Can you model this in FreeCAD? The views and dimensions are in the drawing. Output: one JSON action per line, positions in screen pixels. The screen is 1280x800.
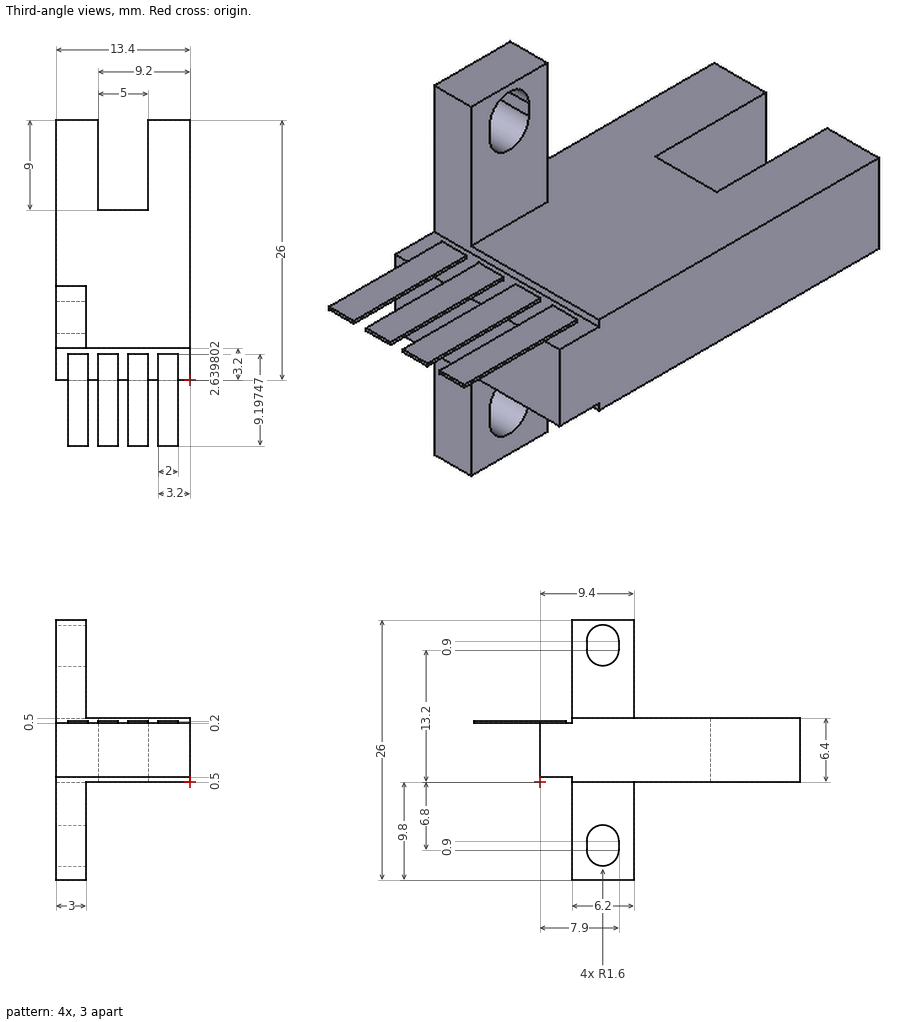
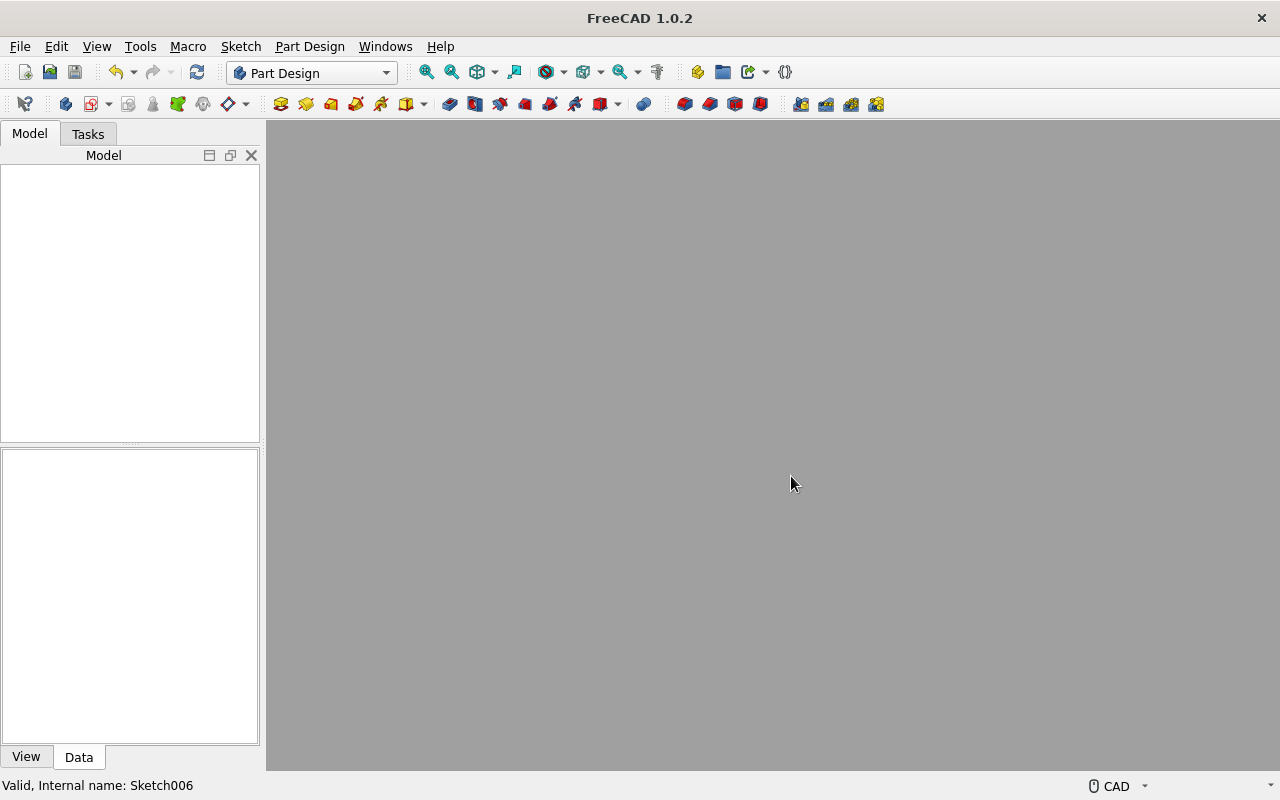
{"action": "left_click", "coordinate": [25, 72]}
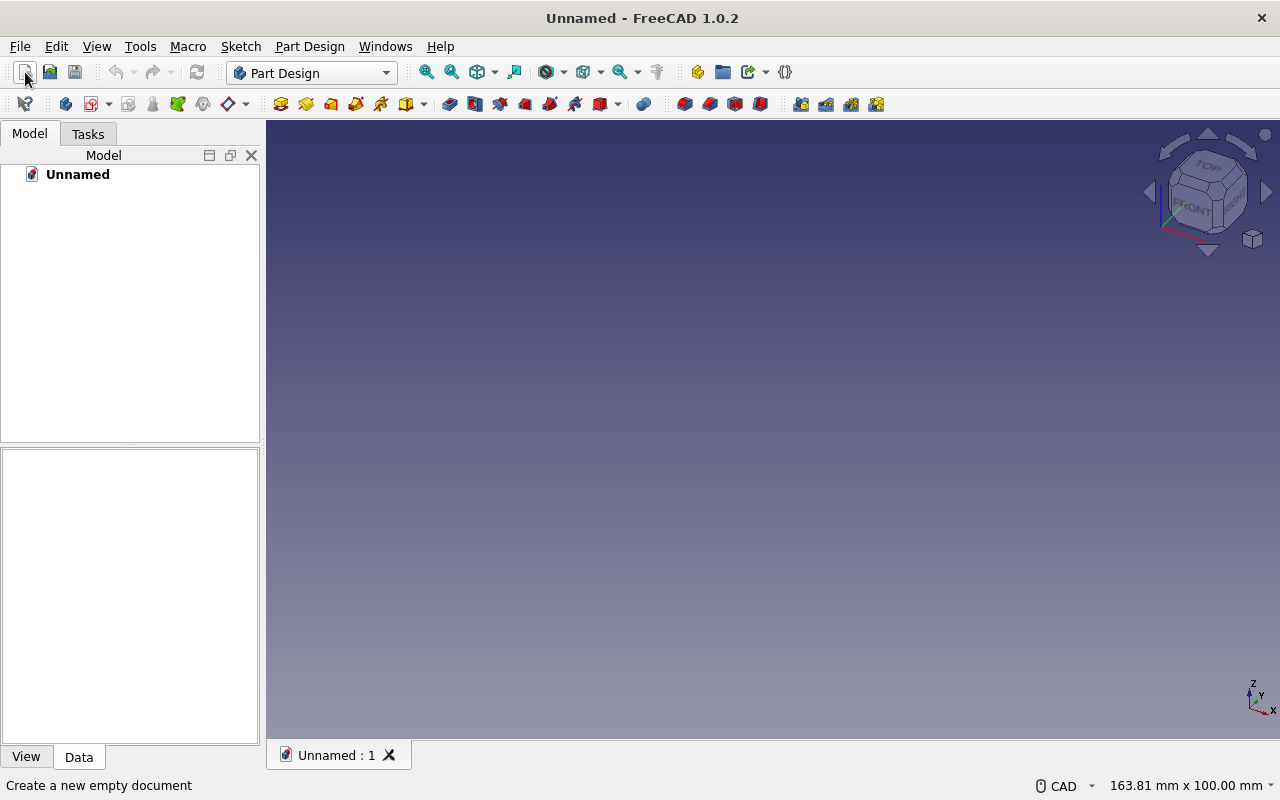
{"action": "left_click", "coordinate": [90, 104]}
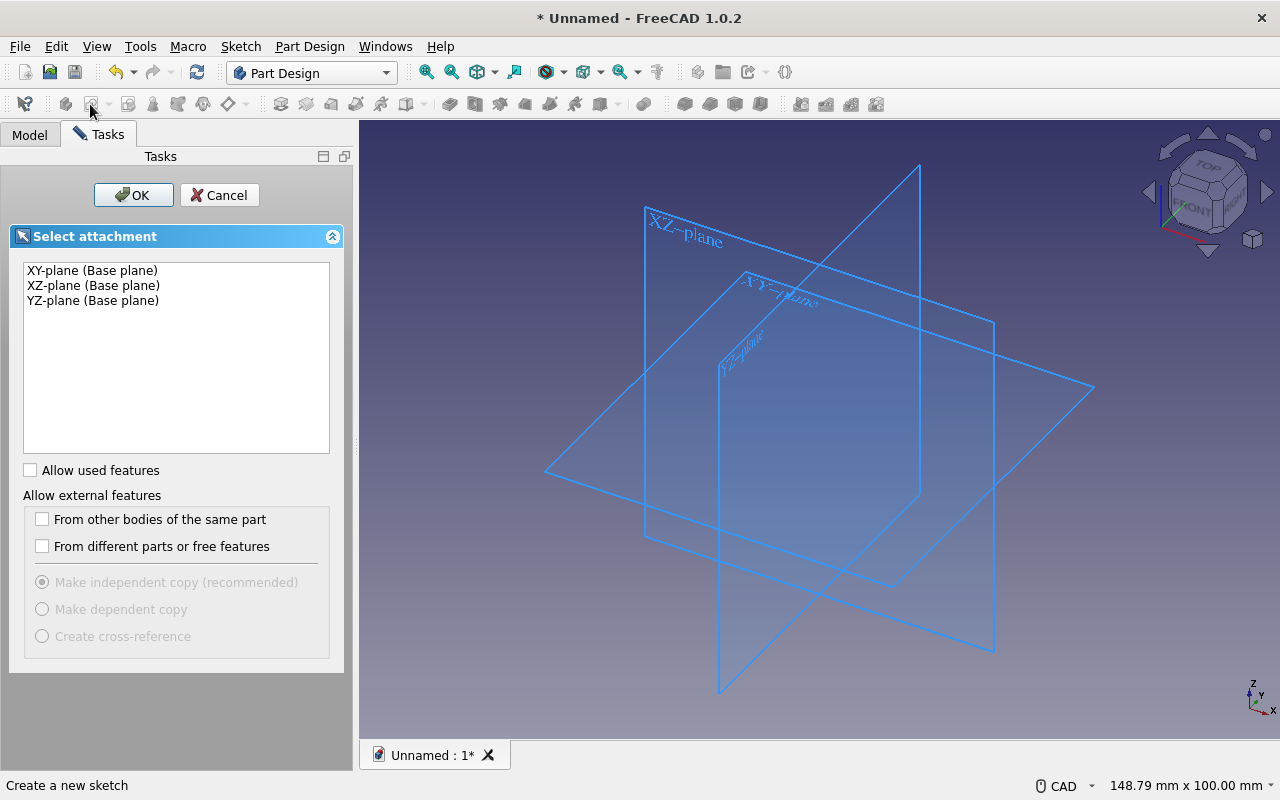
{"action": "left_click", "coordinate": [84, 270]}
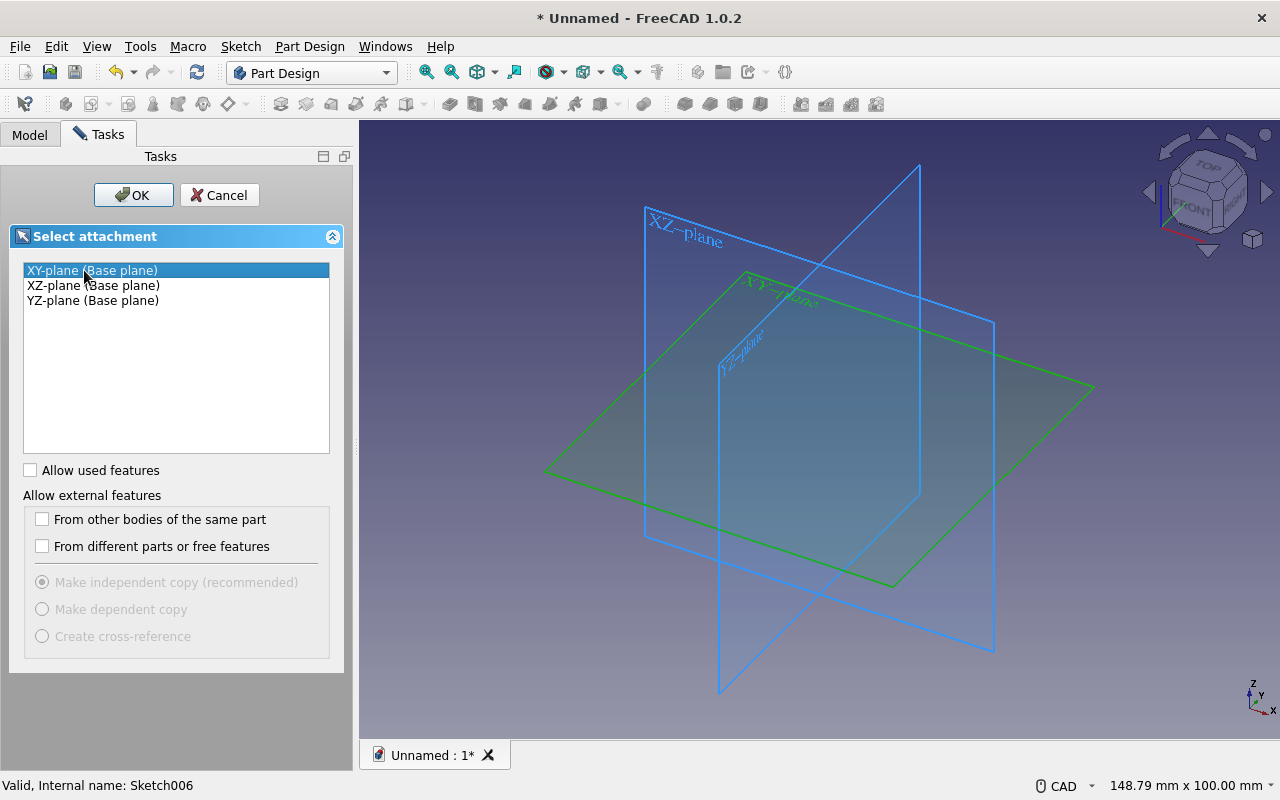
{"action": "left_click", "coordinate": [134, 195]}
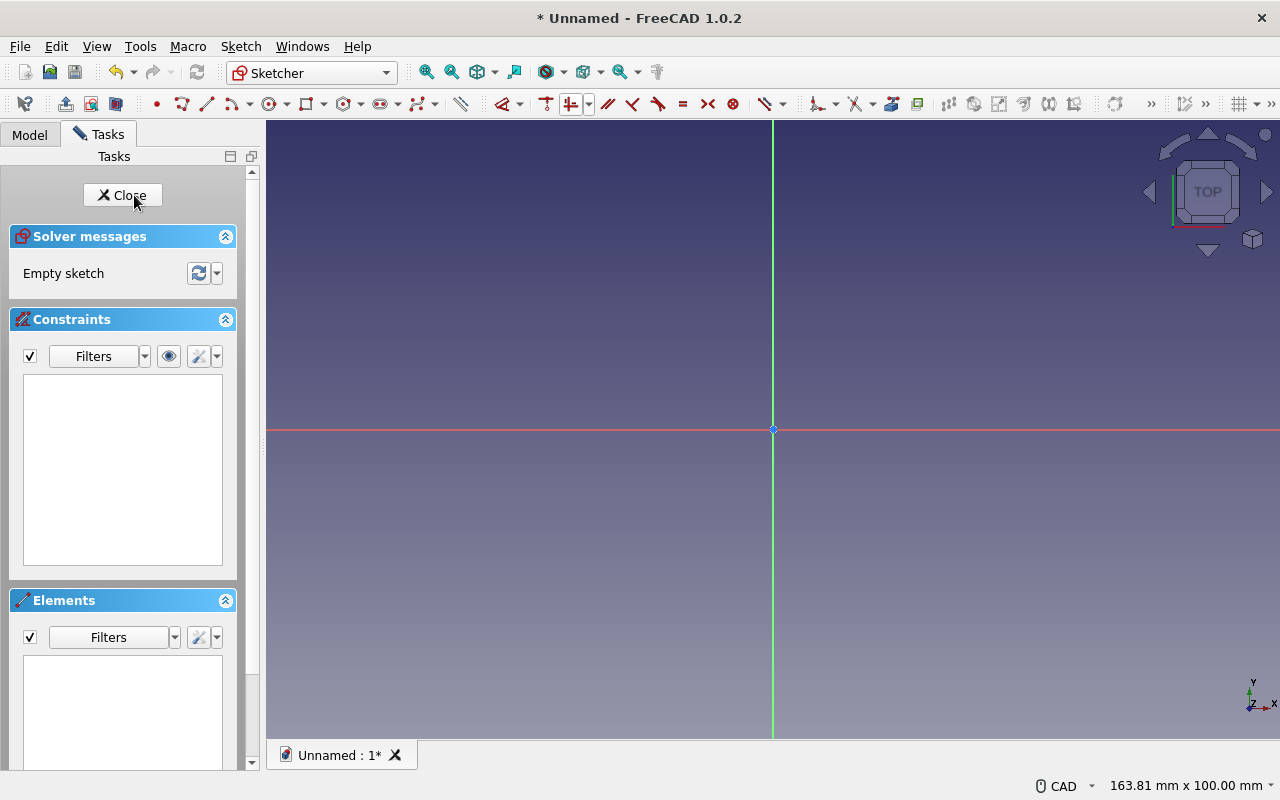
{"action": "scroll", "coordinate": [747, 302], "scroll_direction": "up", "scroll_amount": 5}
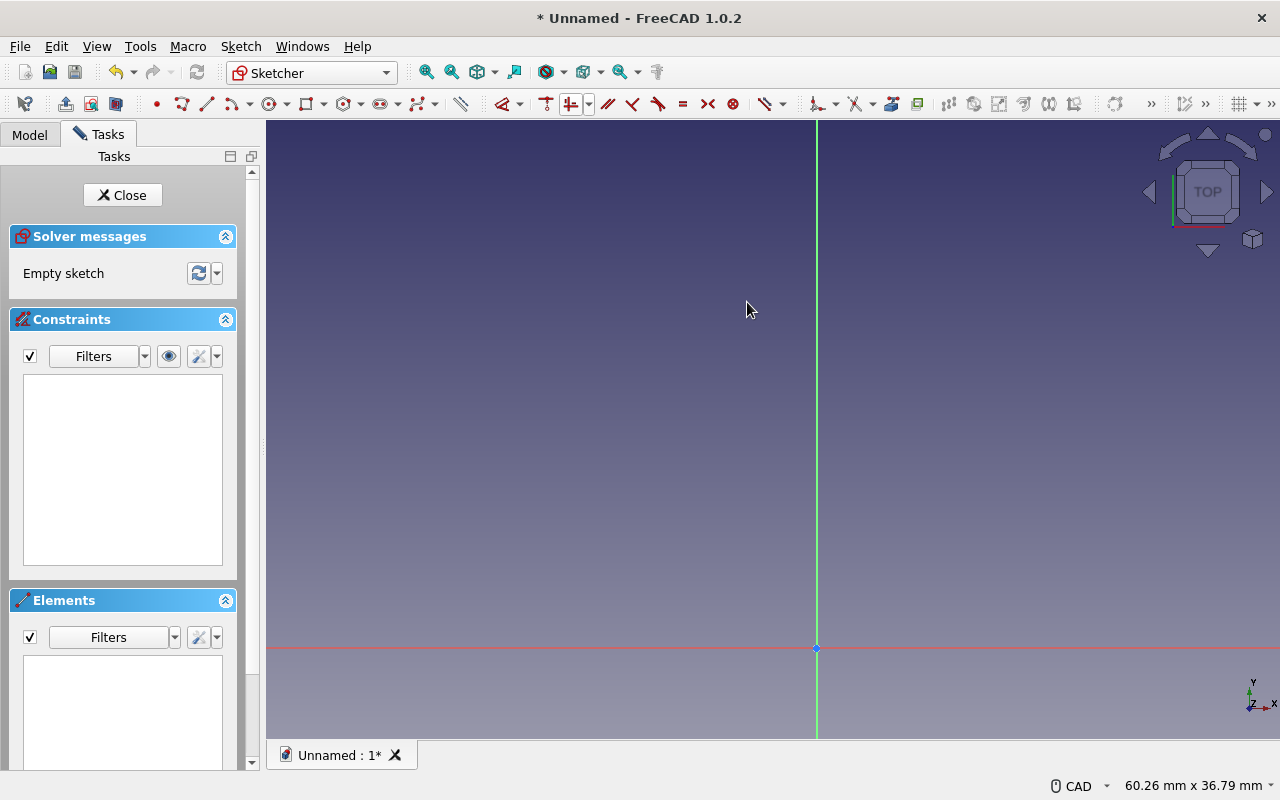
{"action": "left_click", "coordinate": [306, 104]}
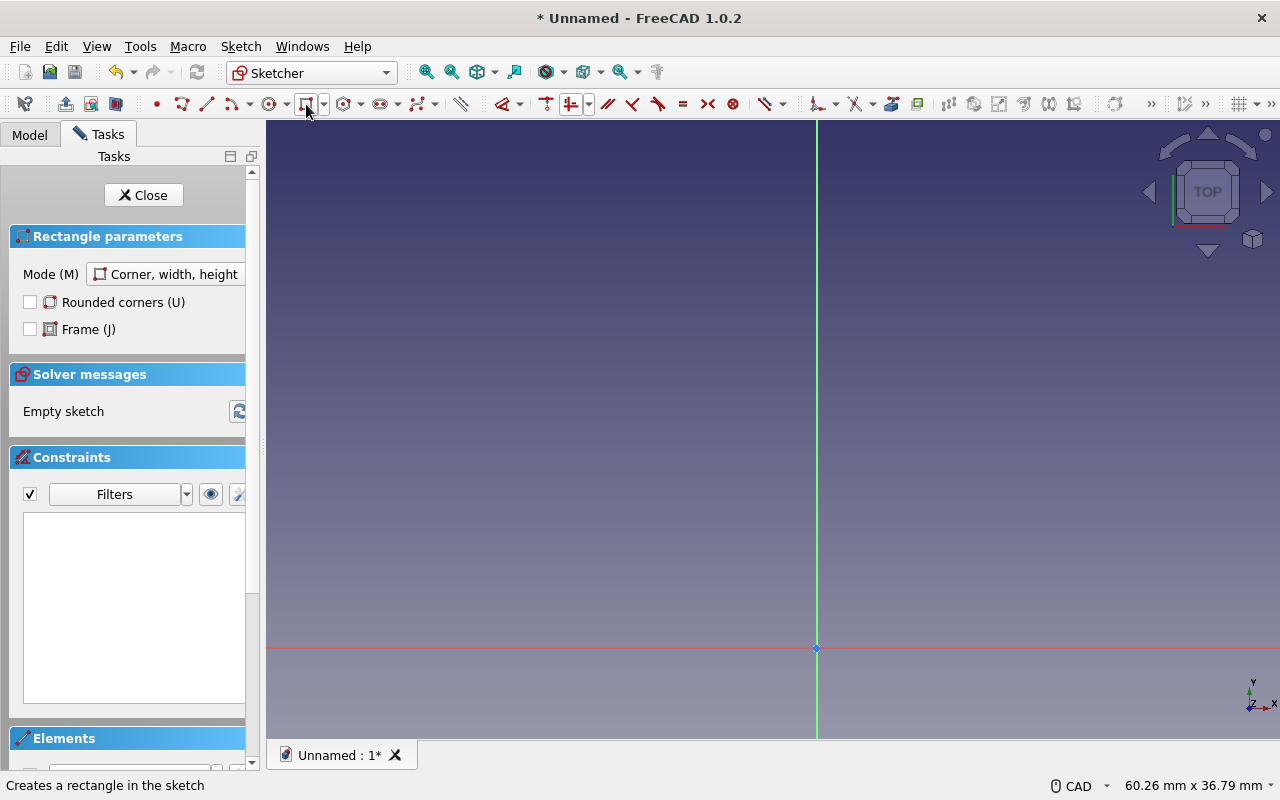
{"action": "left_click", "coordinate": [817, 648]}
{"action": "left_click", "coordinate": [591, 211]}
{"action": "key", "text": "Escape"}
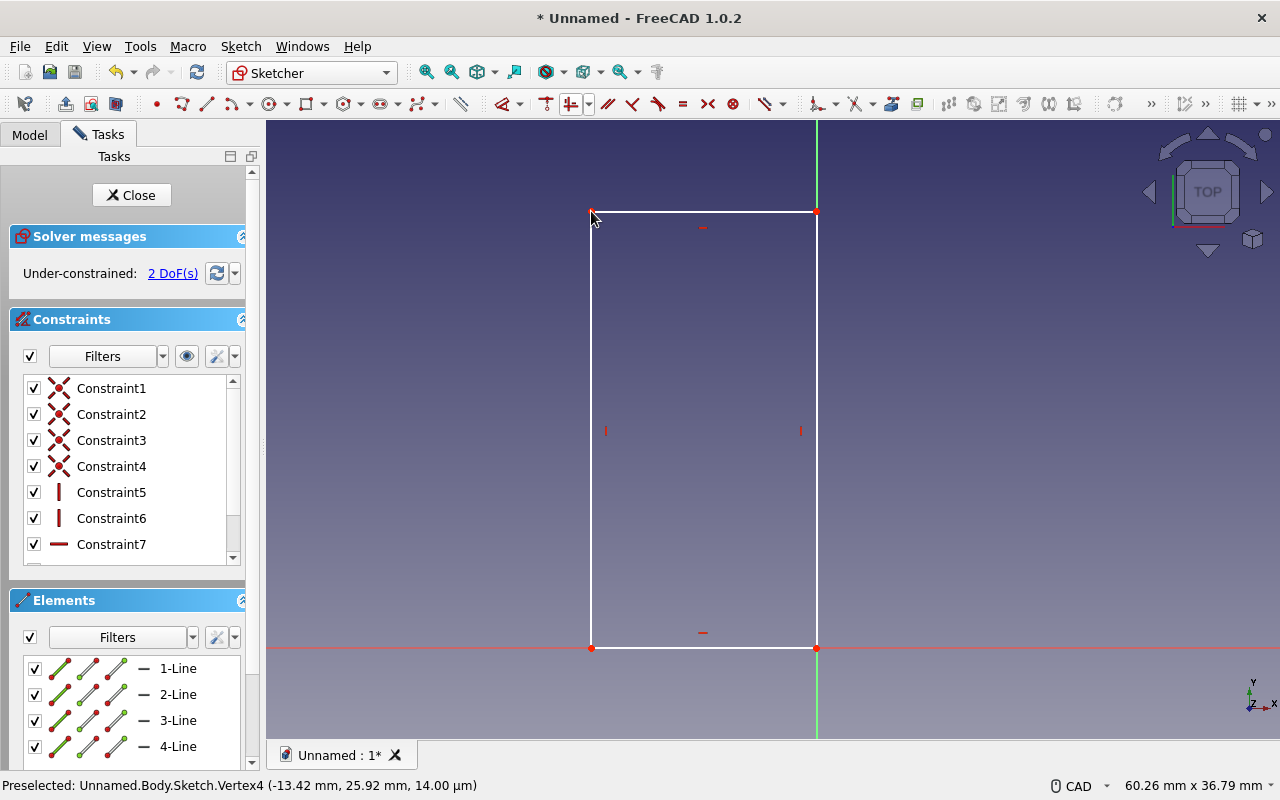
{"action": "left_click", "coordinate": [502, 104]}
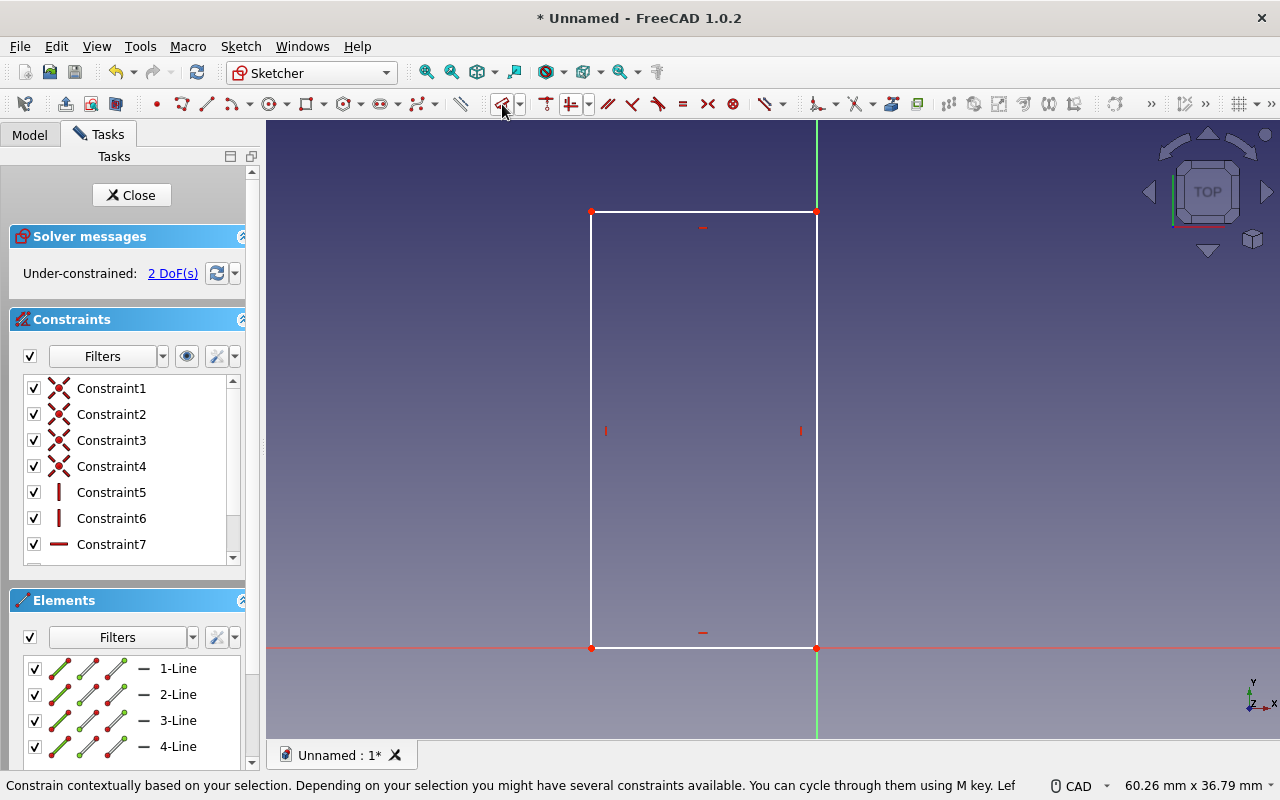
{"action": "left_click", "coordinate": [817, 517]}
{"action": "left_click", "coordinate": [851, 430]}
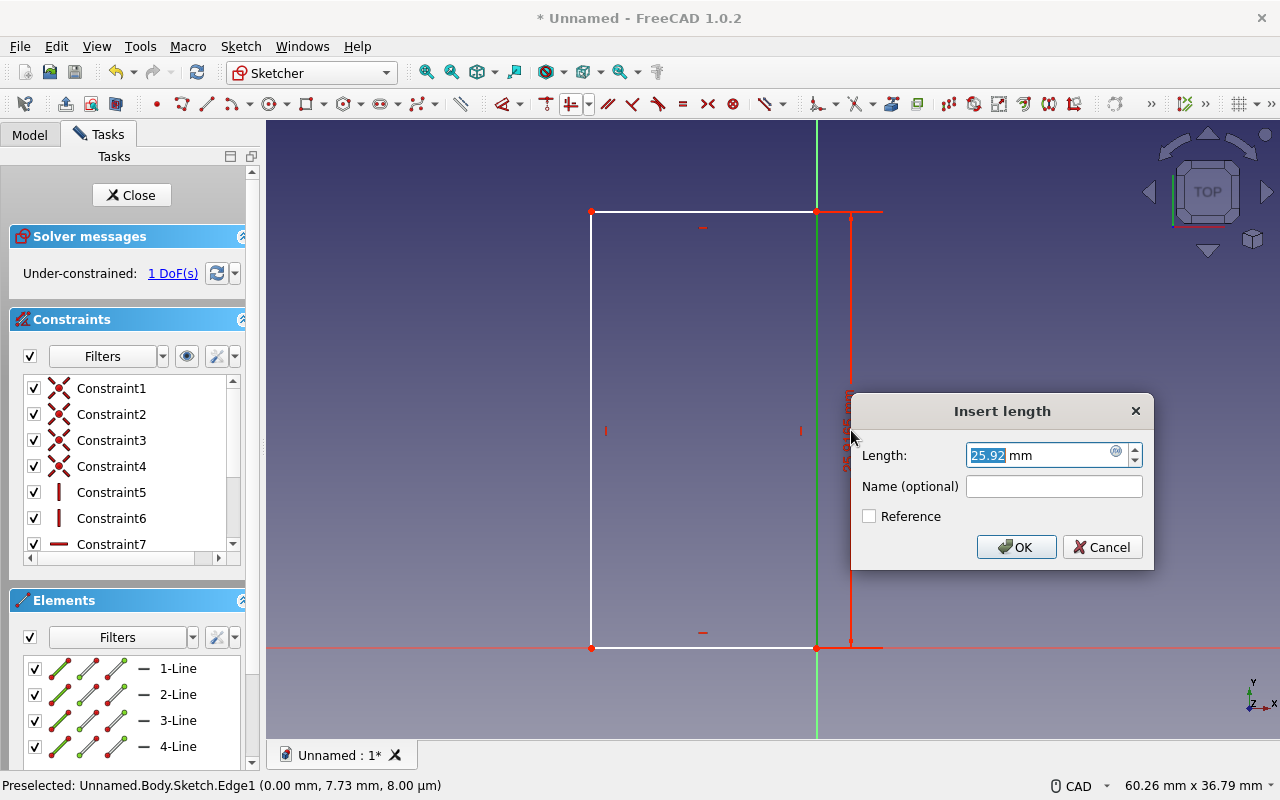
{"action": "type", "text": "26"}
{"action": "key", "text": "Return"}